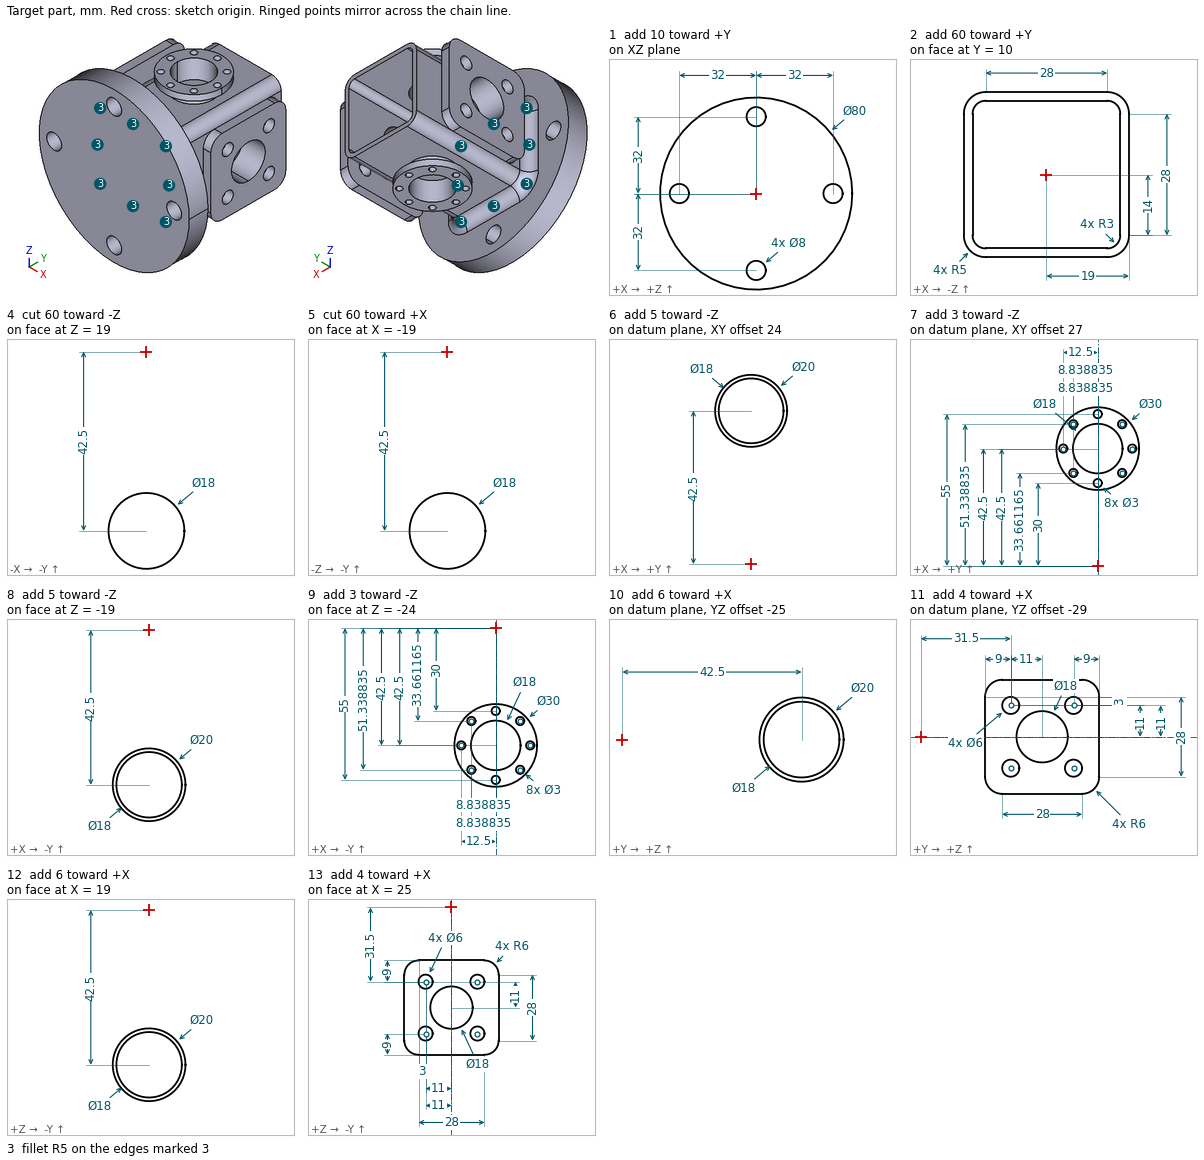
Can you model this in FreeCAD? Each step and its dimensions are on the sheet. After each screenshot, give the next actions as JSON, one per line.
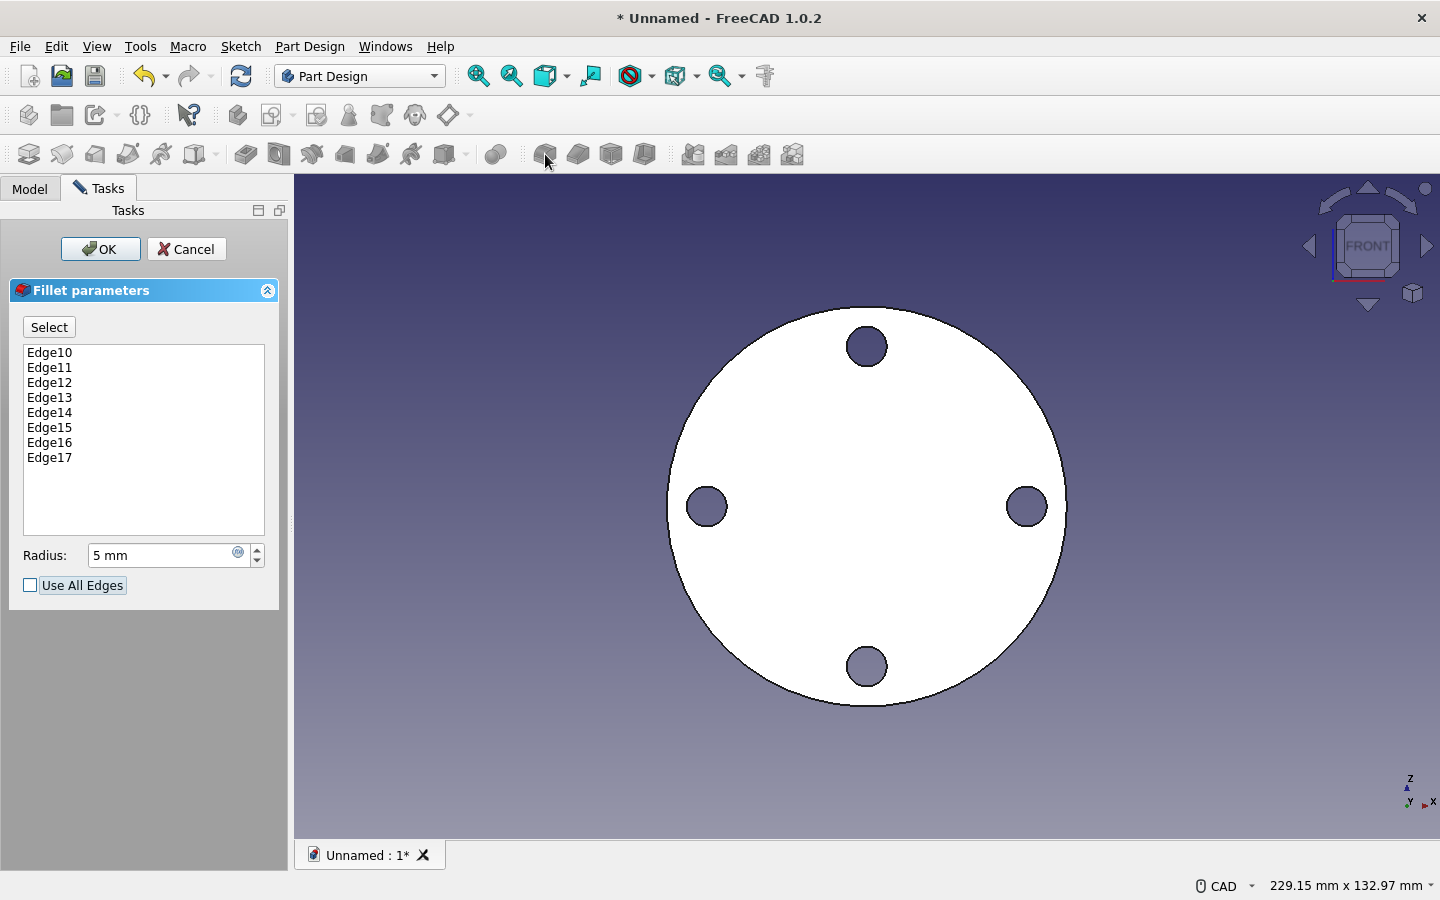
{"action": "left_click", "coordinate": [101, 249]}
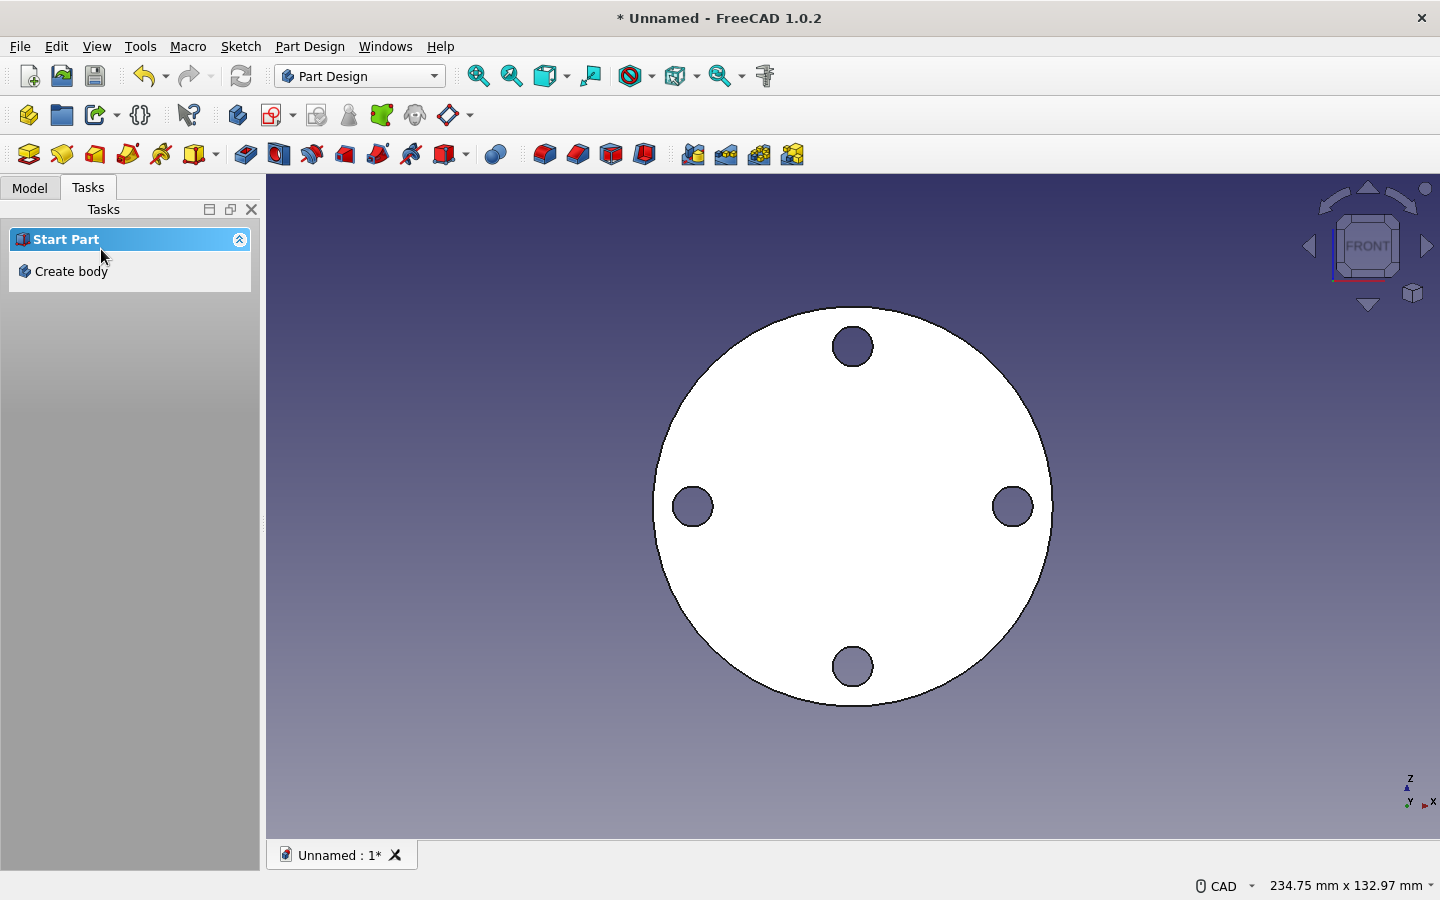
{"action": "key", "text": "0"}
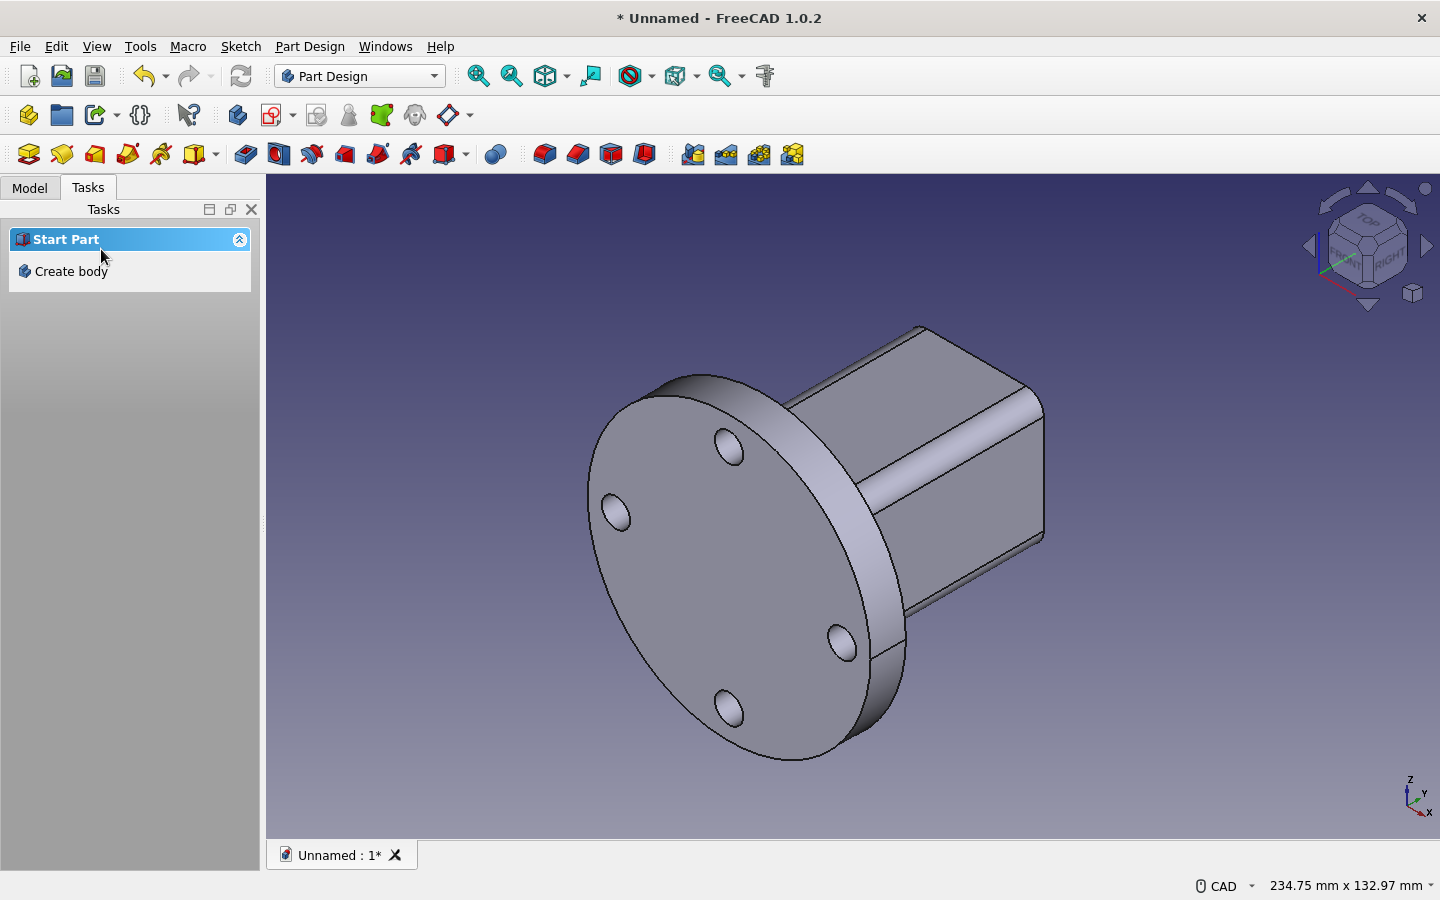
{"action": "left_click", "coordinate": [907, 396]}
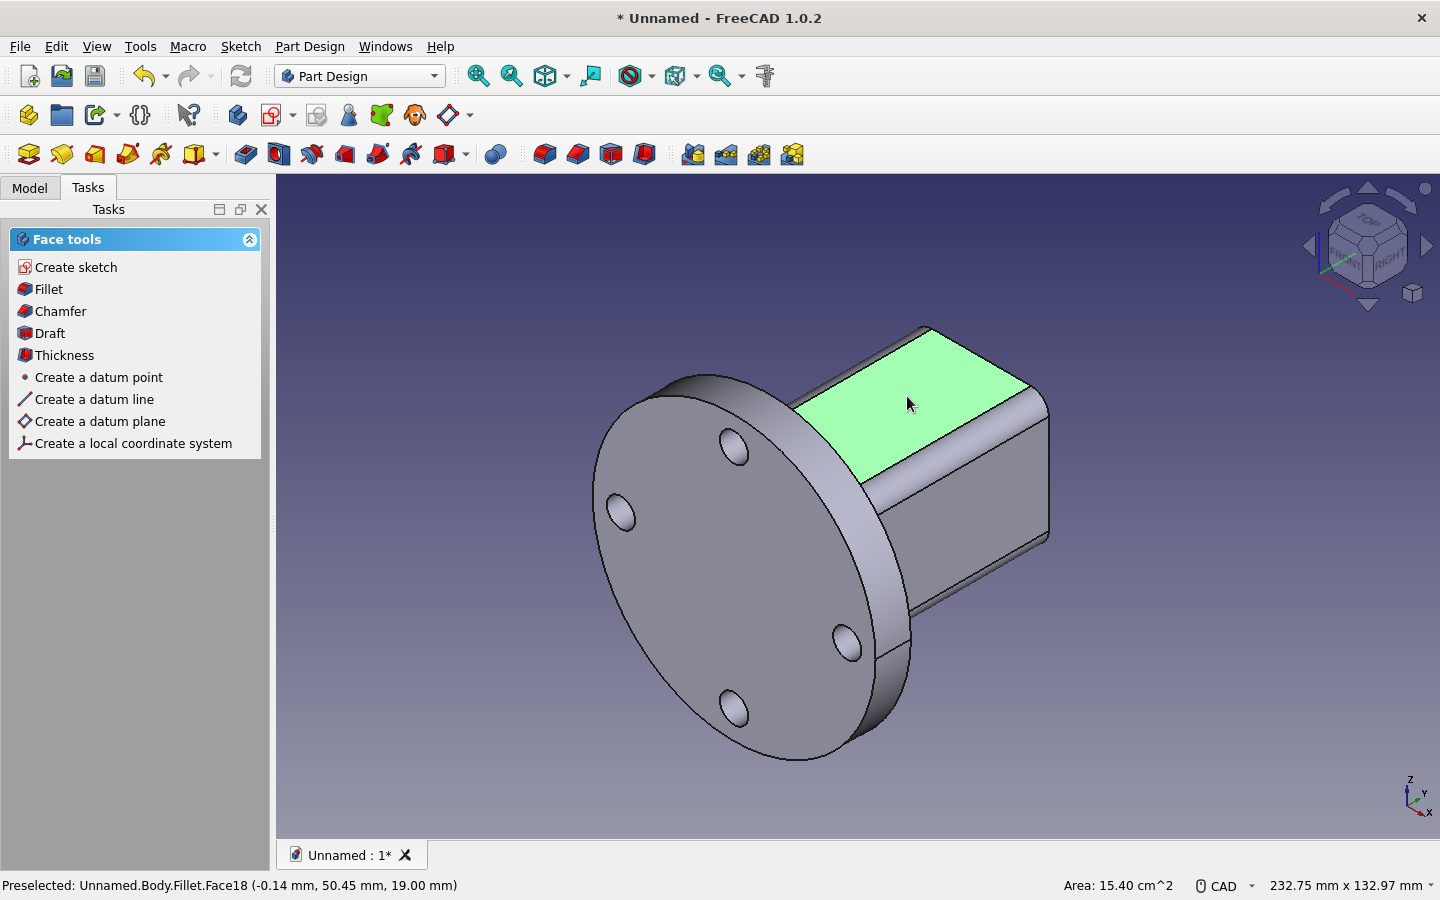
{"action": "left_click", "coordinate": [270, 116]}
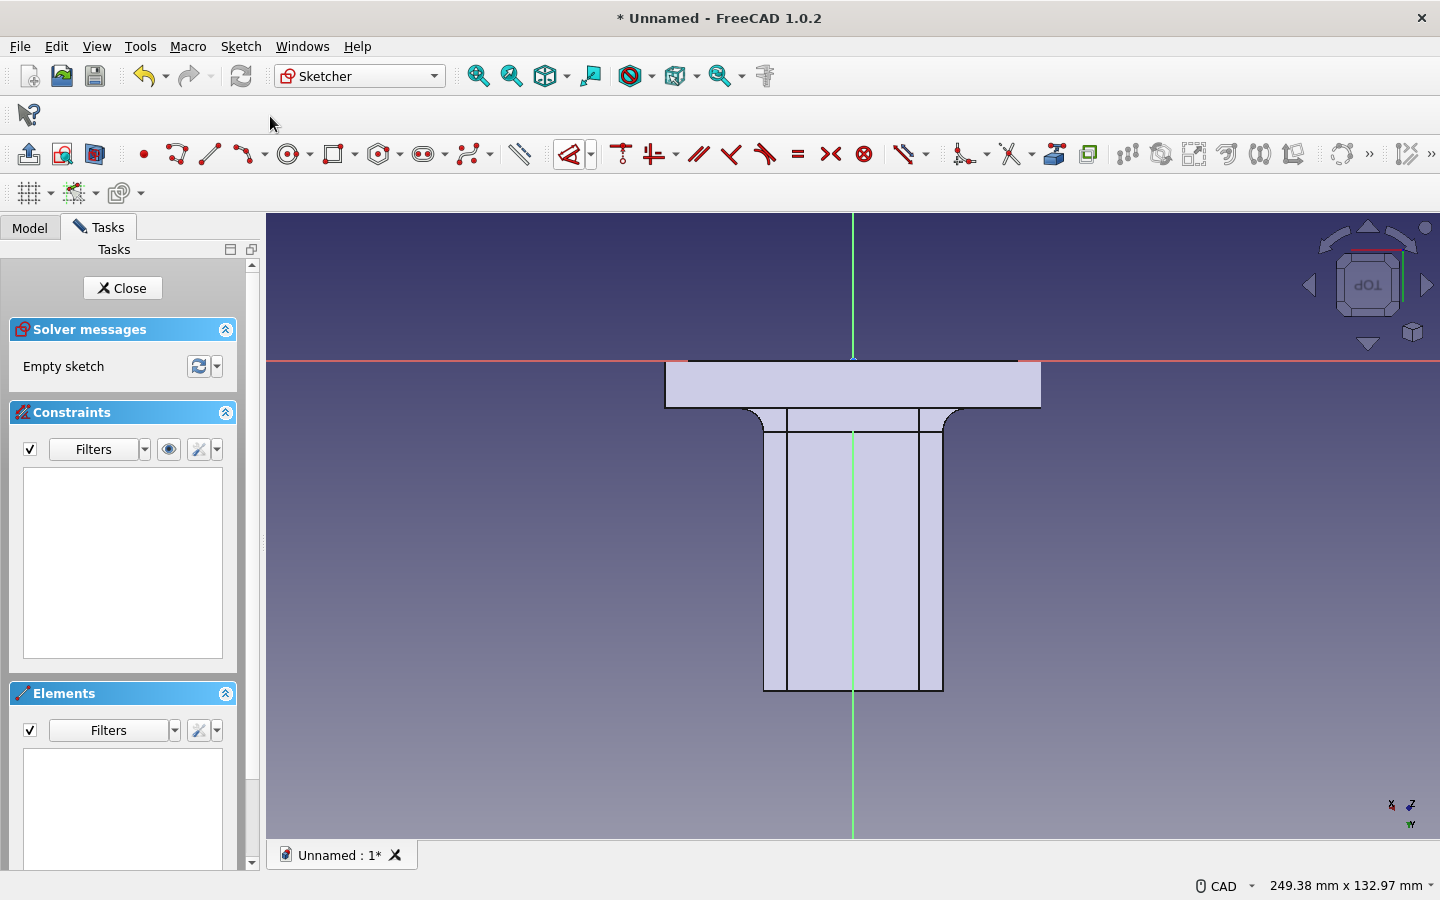
{"action": "key", "text": "q s"}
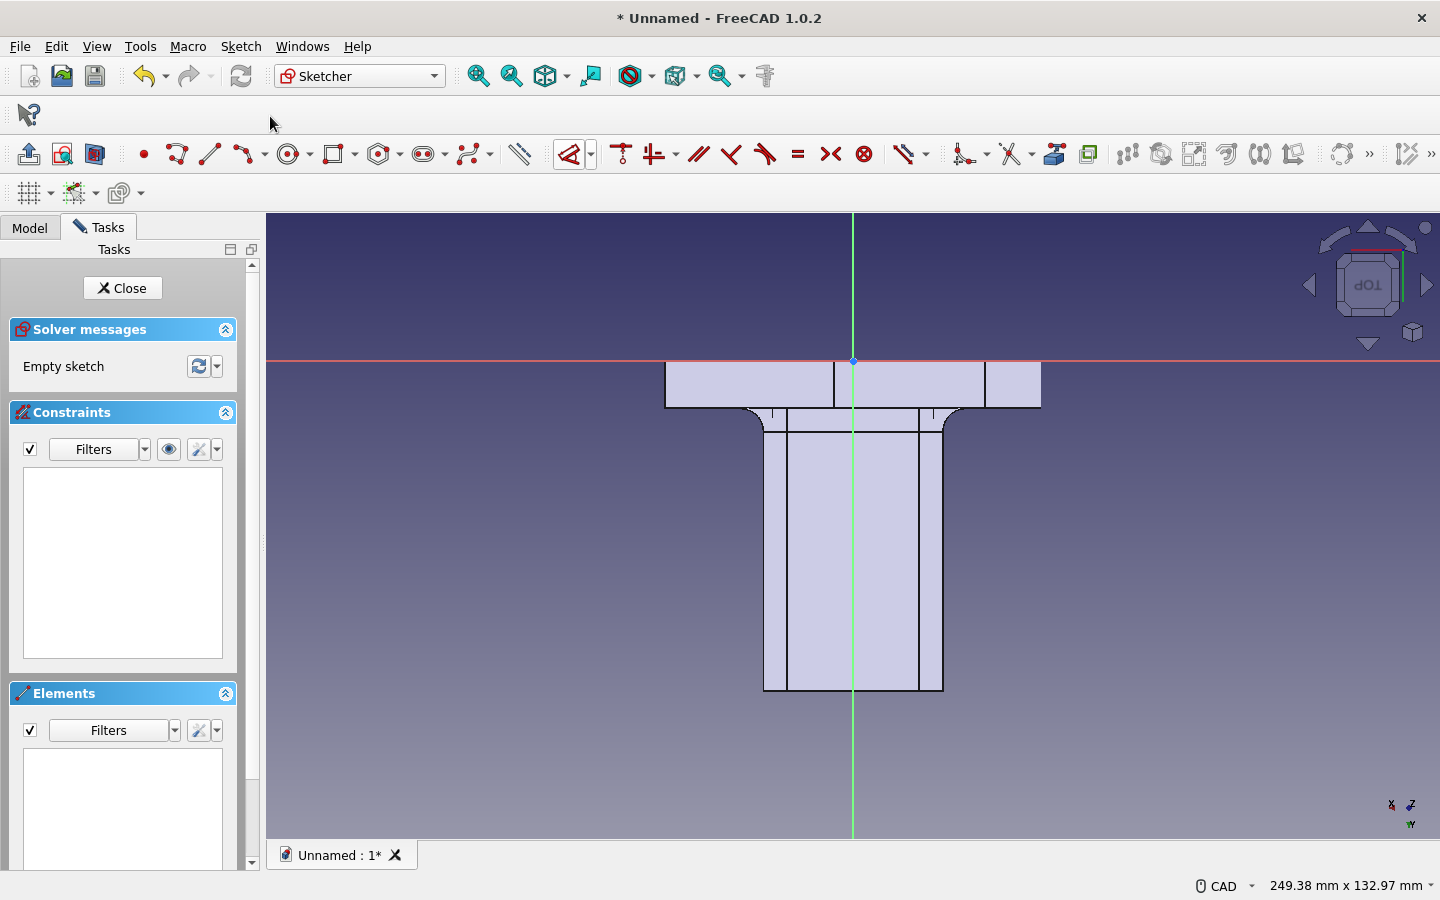
{"action": "scroll", "coordinate": [871, 570], "scroll_direction": "up", "scroll_amount": 8}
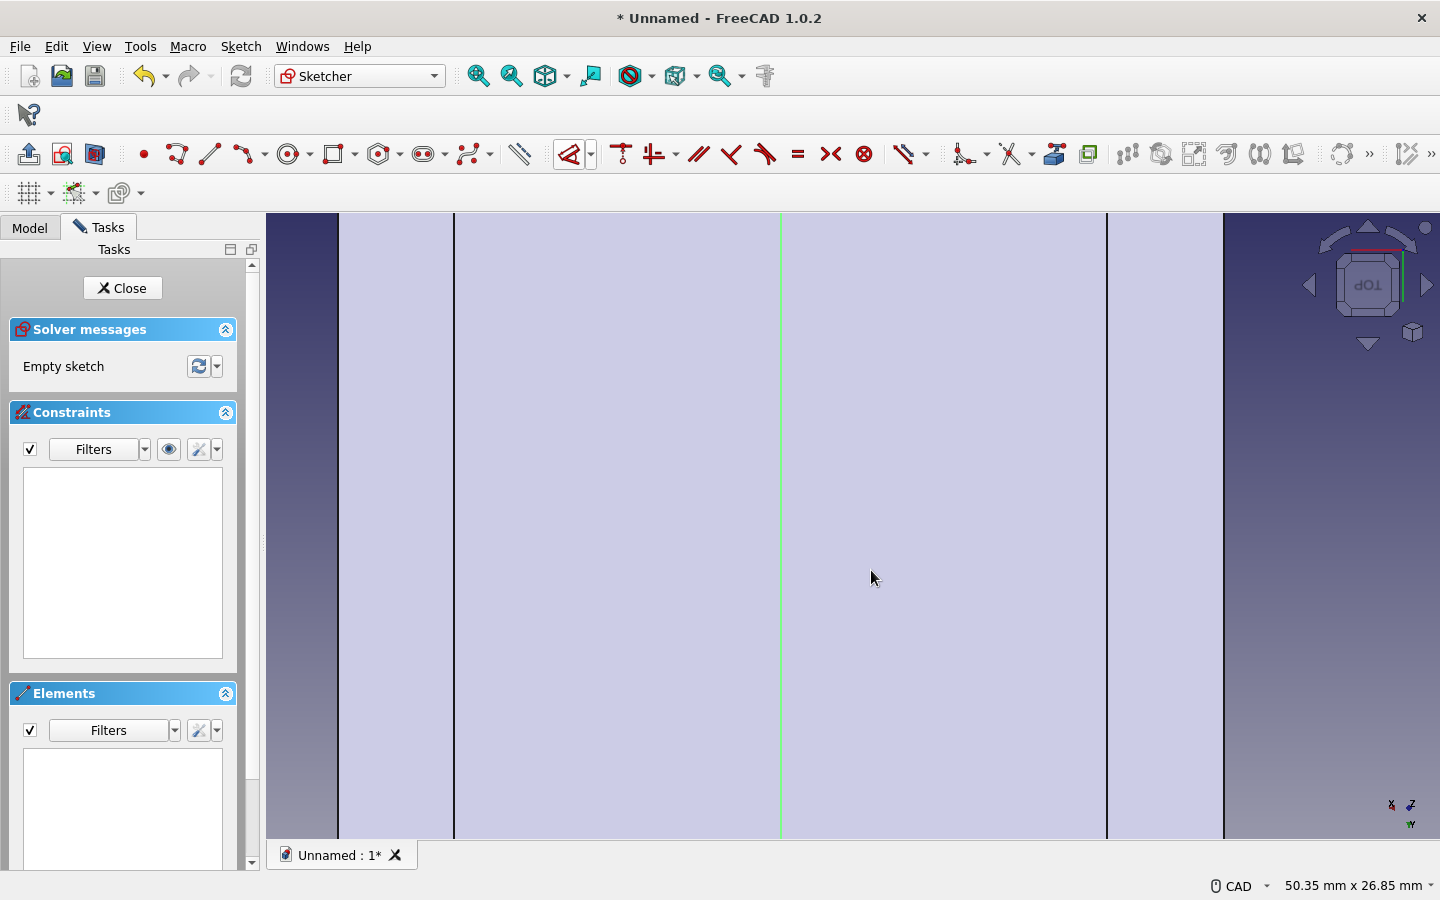
{"action": "left_click", "coordinate": [288, 154]}